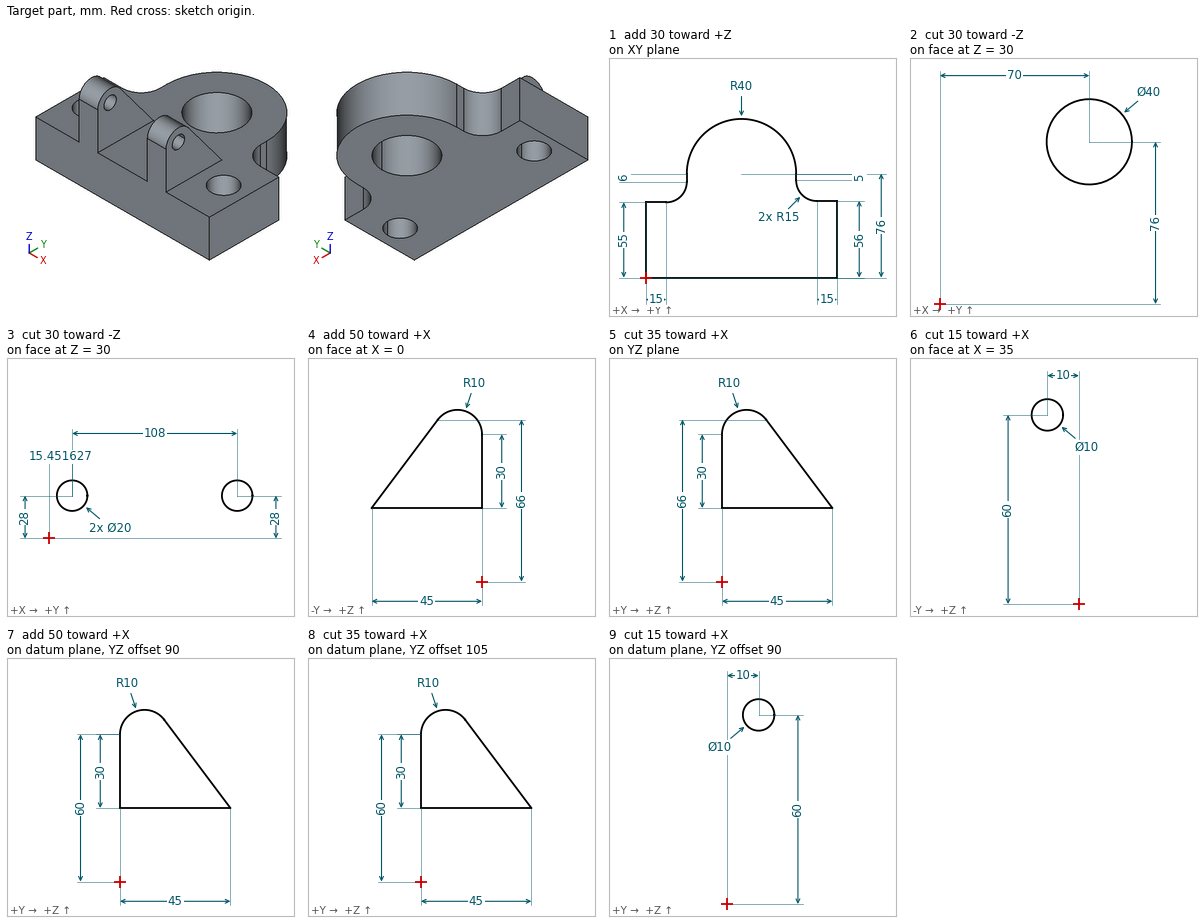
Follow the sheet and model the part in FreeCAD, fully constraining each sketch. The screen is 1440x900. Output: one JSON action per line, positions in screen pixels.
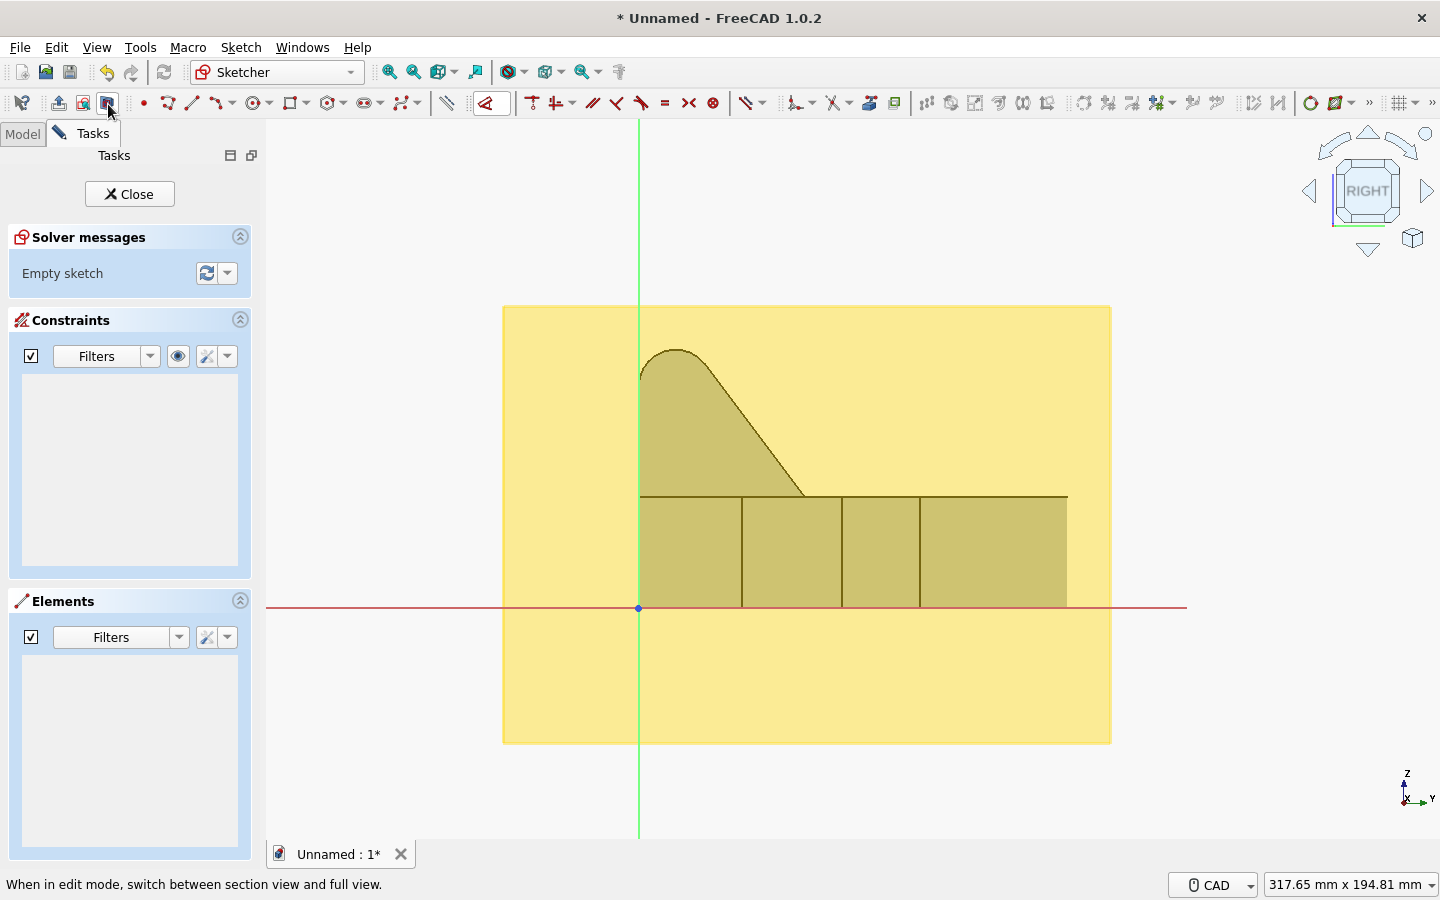
{"action": "scroll", "coordinate": [646, 481], "scroll_direction": "up", "scroll_amount": 3}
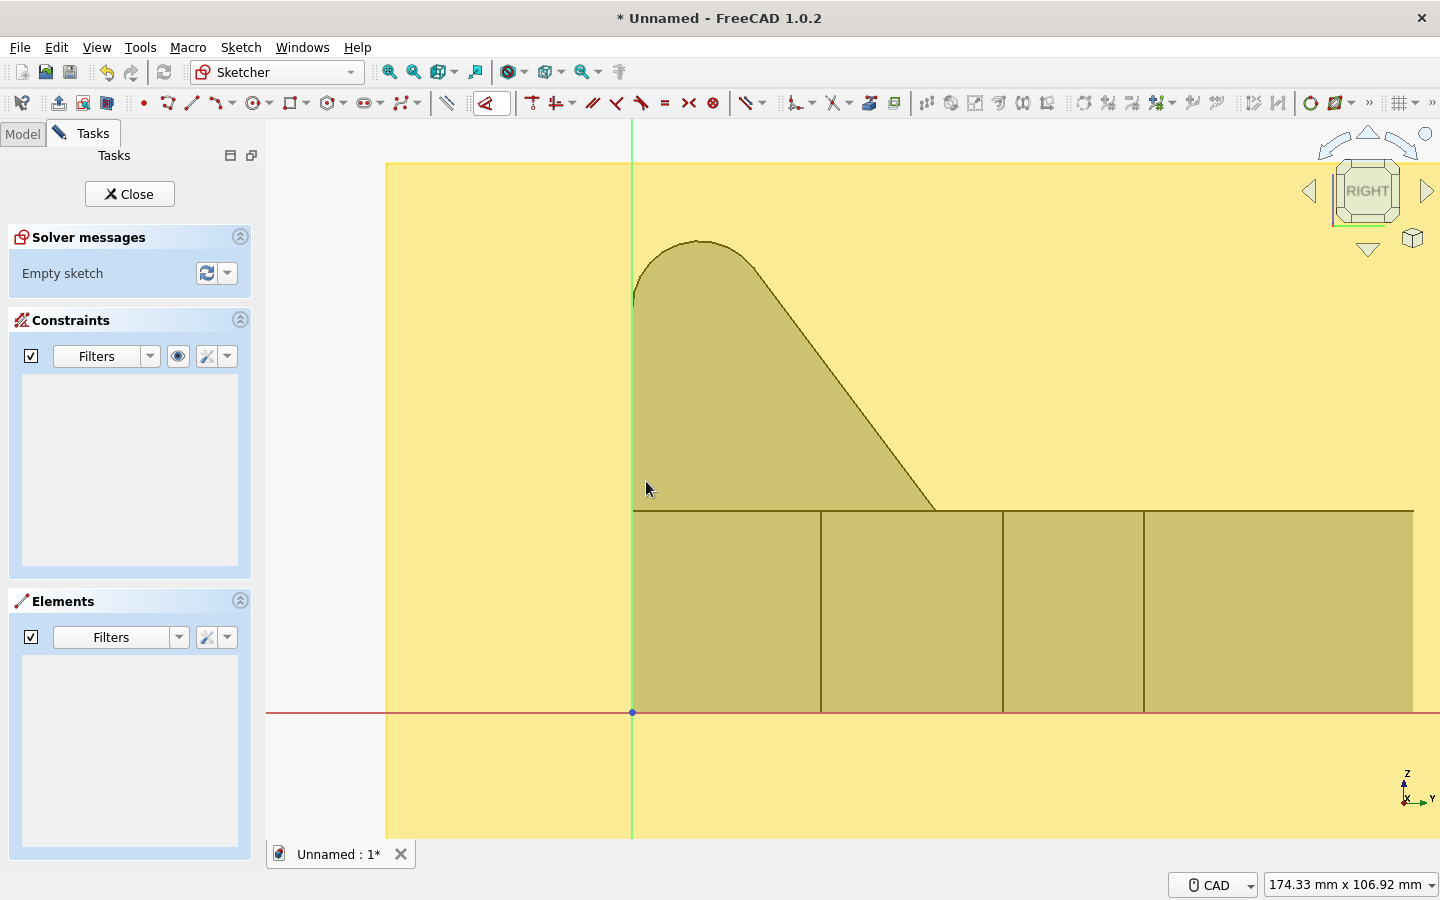
{"action": "key", "text": "g m"}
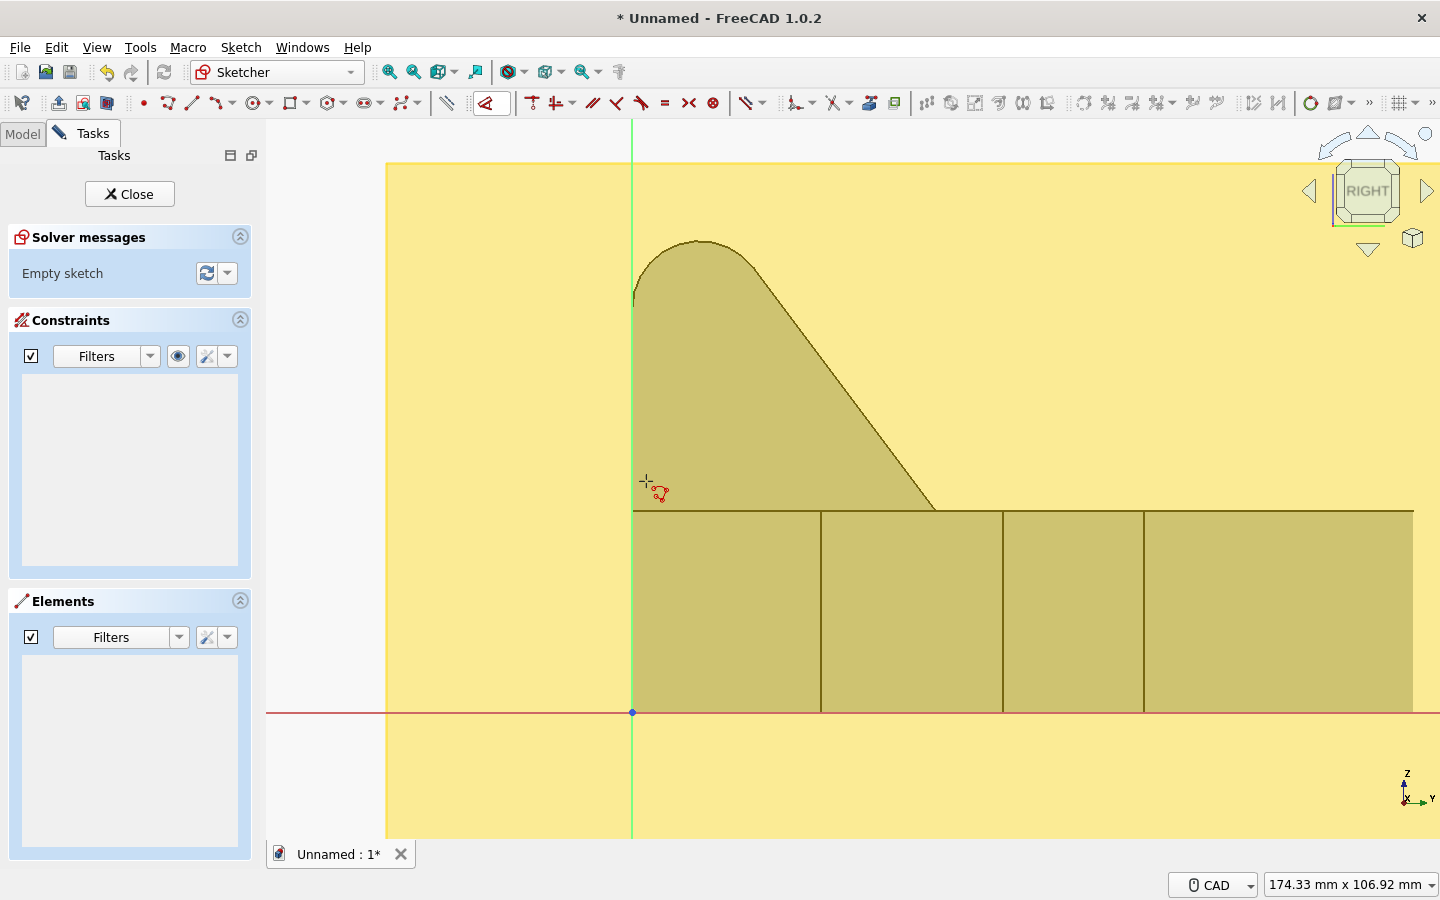
{"action": "left_click", "coordinate": [632, 308]}
{"action": "left_click", "coordinate": [641, 511]}
{"action": "left_click", "coordinate": [935, 511]}
{"action": "left_click", "coordinate": [754, 268]}
{"action": "right_click", "coordinate": [754, 268]}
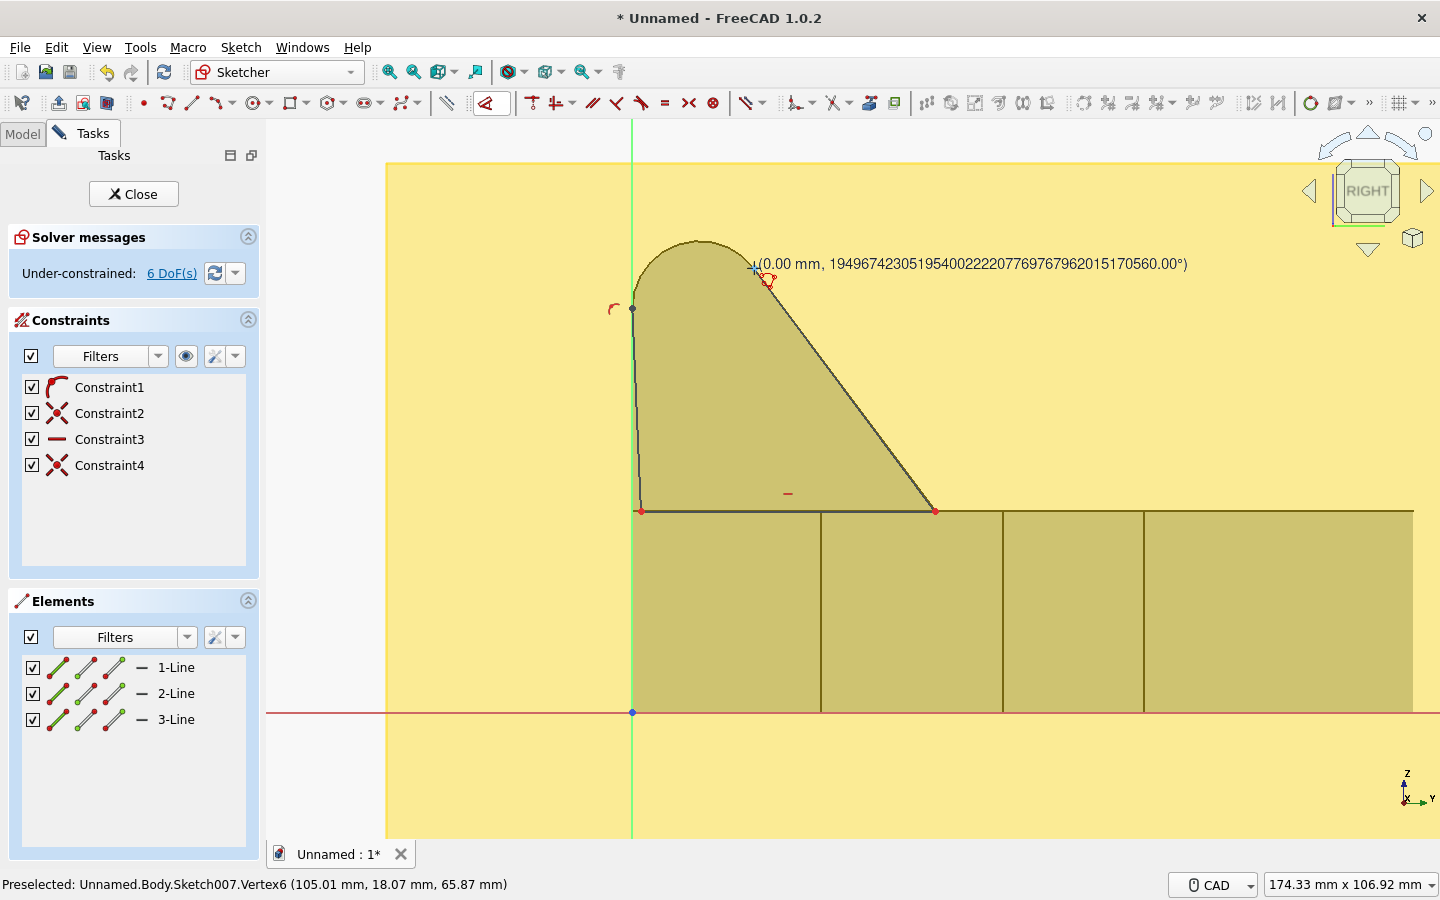
{"action": "left_click", "coordinate": [216, 104]}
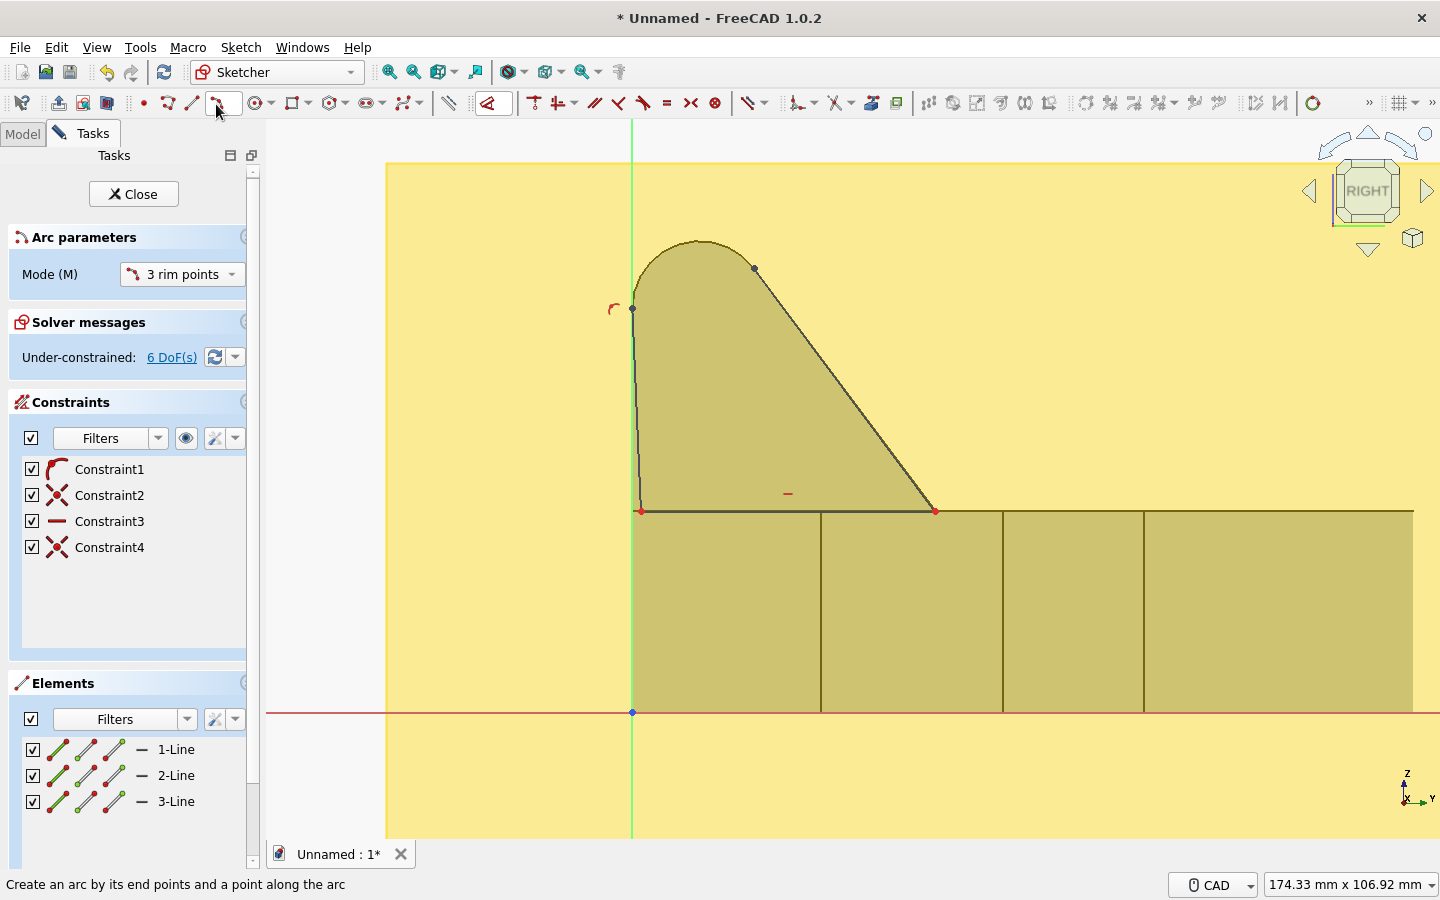
{"action": "left_click", "coordinate": [754, 269]}
{"action": "left_click", "coordinate": [632, 309]}
{"action": "left_click", "coordinate": [678, 245]}
{"action": "key", "text": "Escape"}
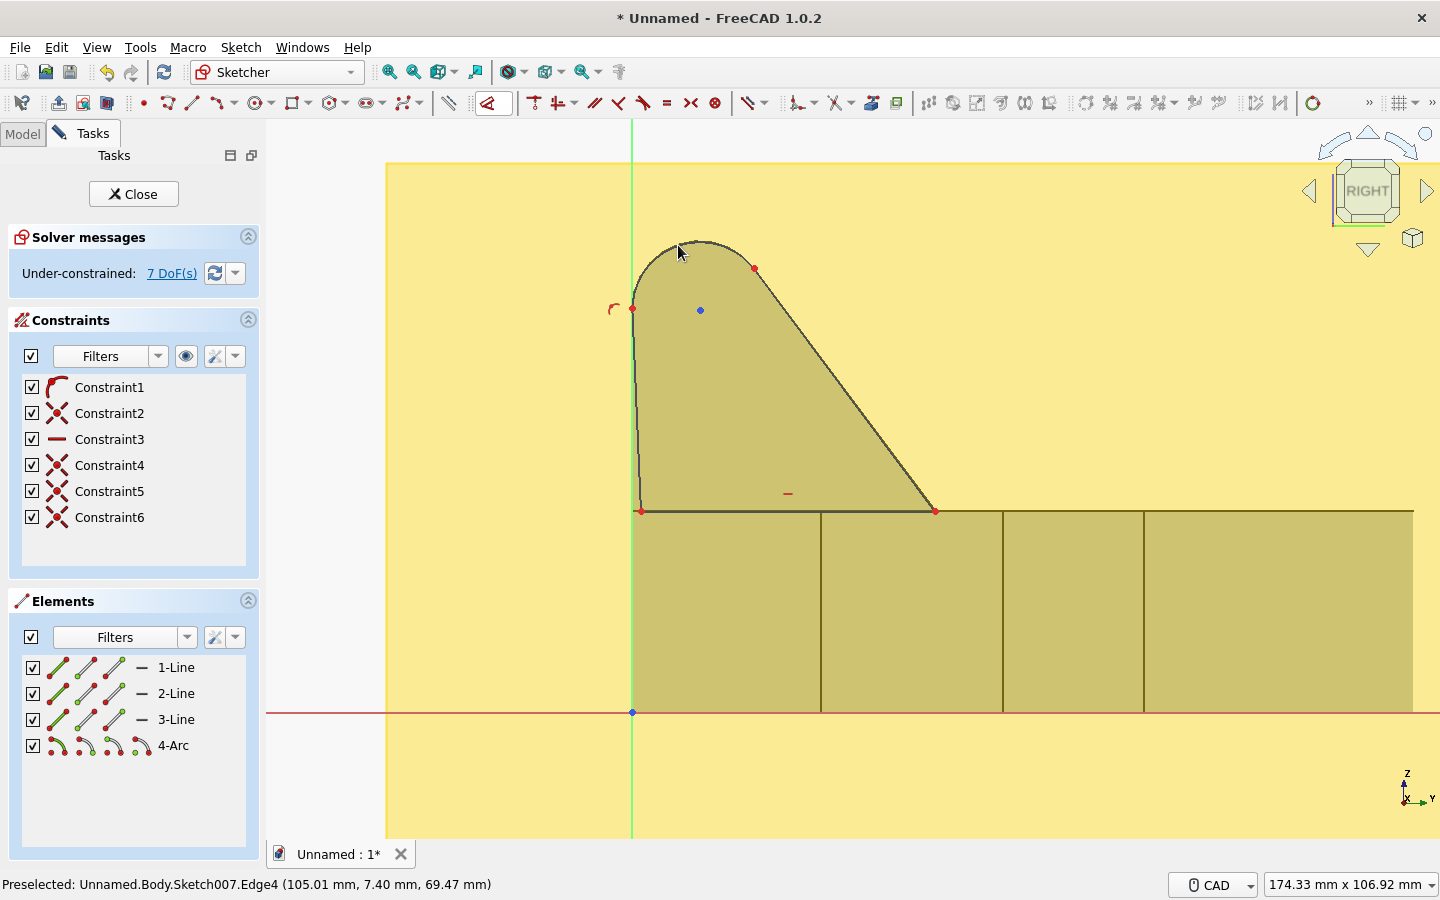
{"action": "left_click", "coordinate": [635, 370]}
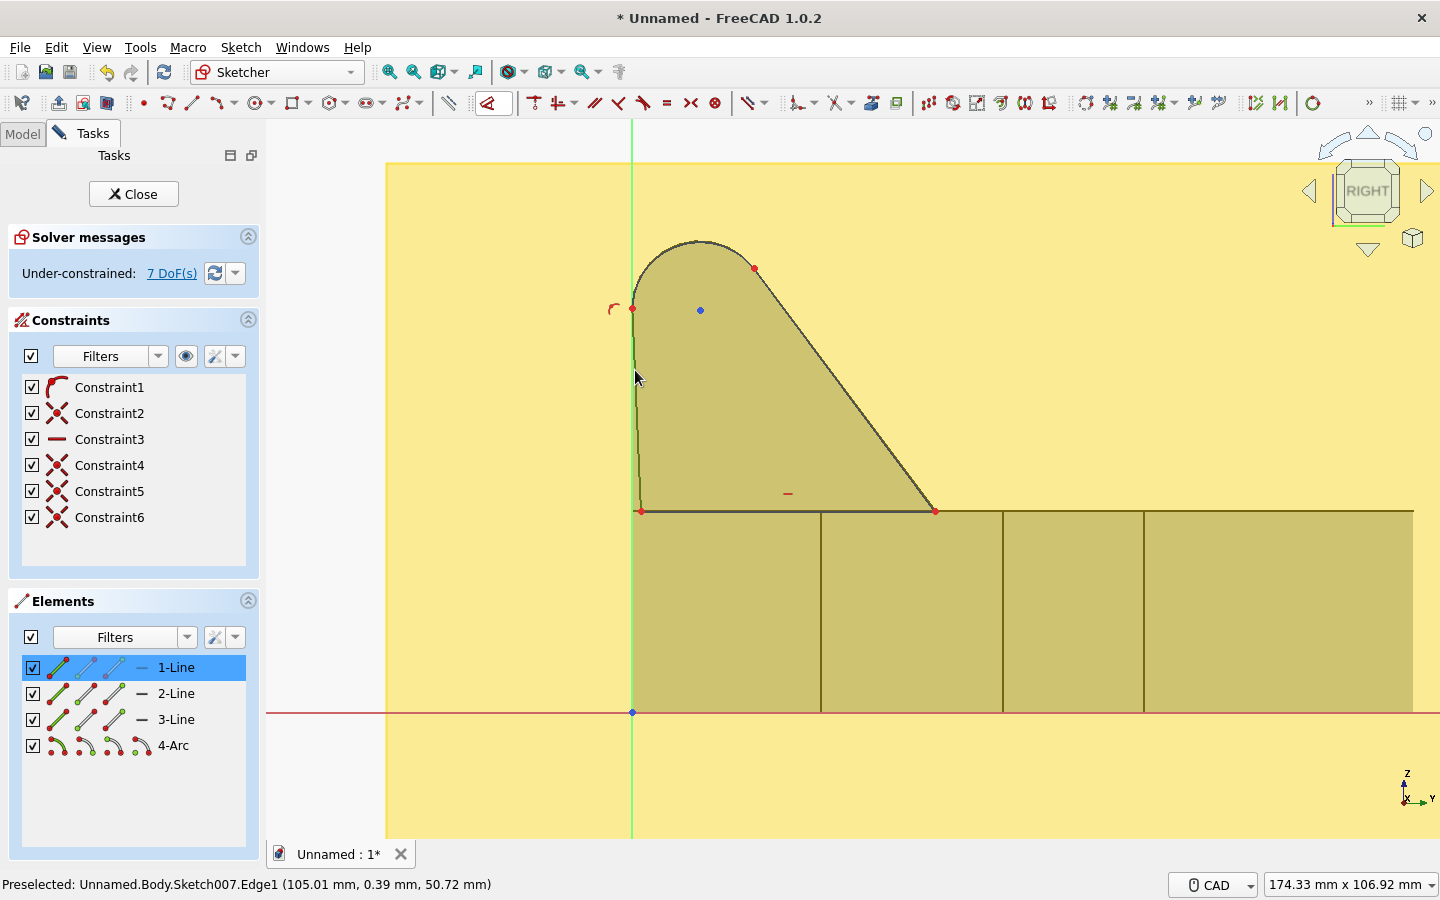
{"action": "left_click", "coordinate": [712, 243]}